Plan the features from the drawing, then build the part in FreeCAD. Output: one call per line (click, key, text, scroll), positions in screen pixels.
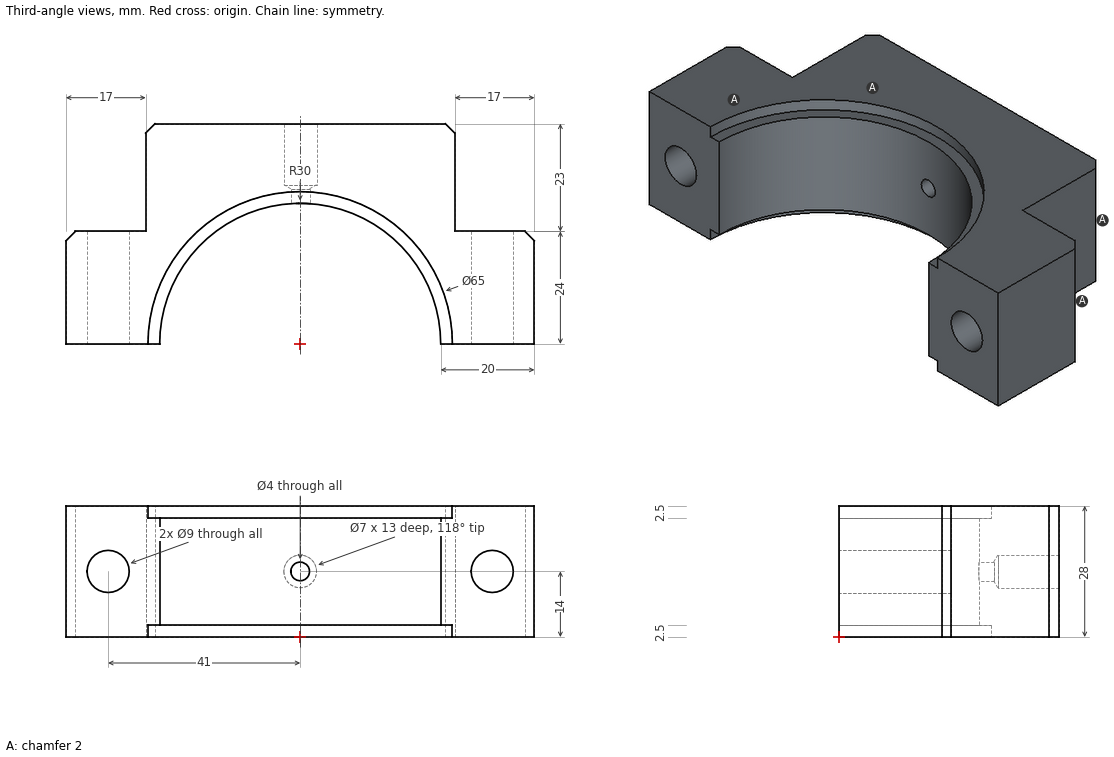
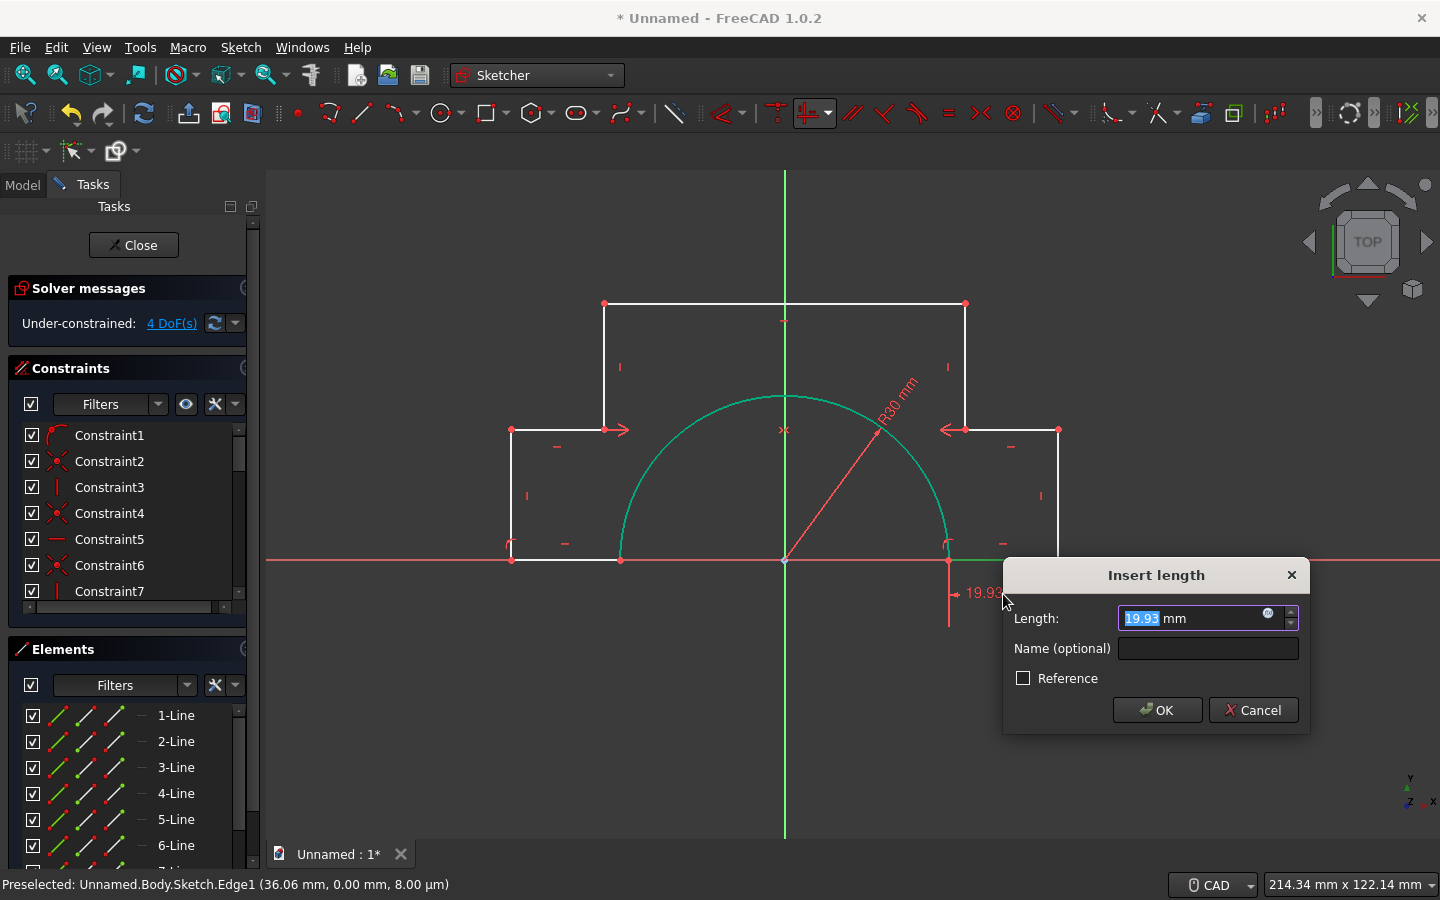
text(20)
key(Return)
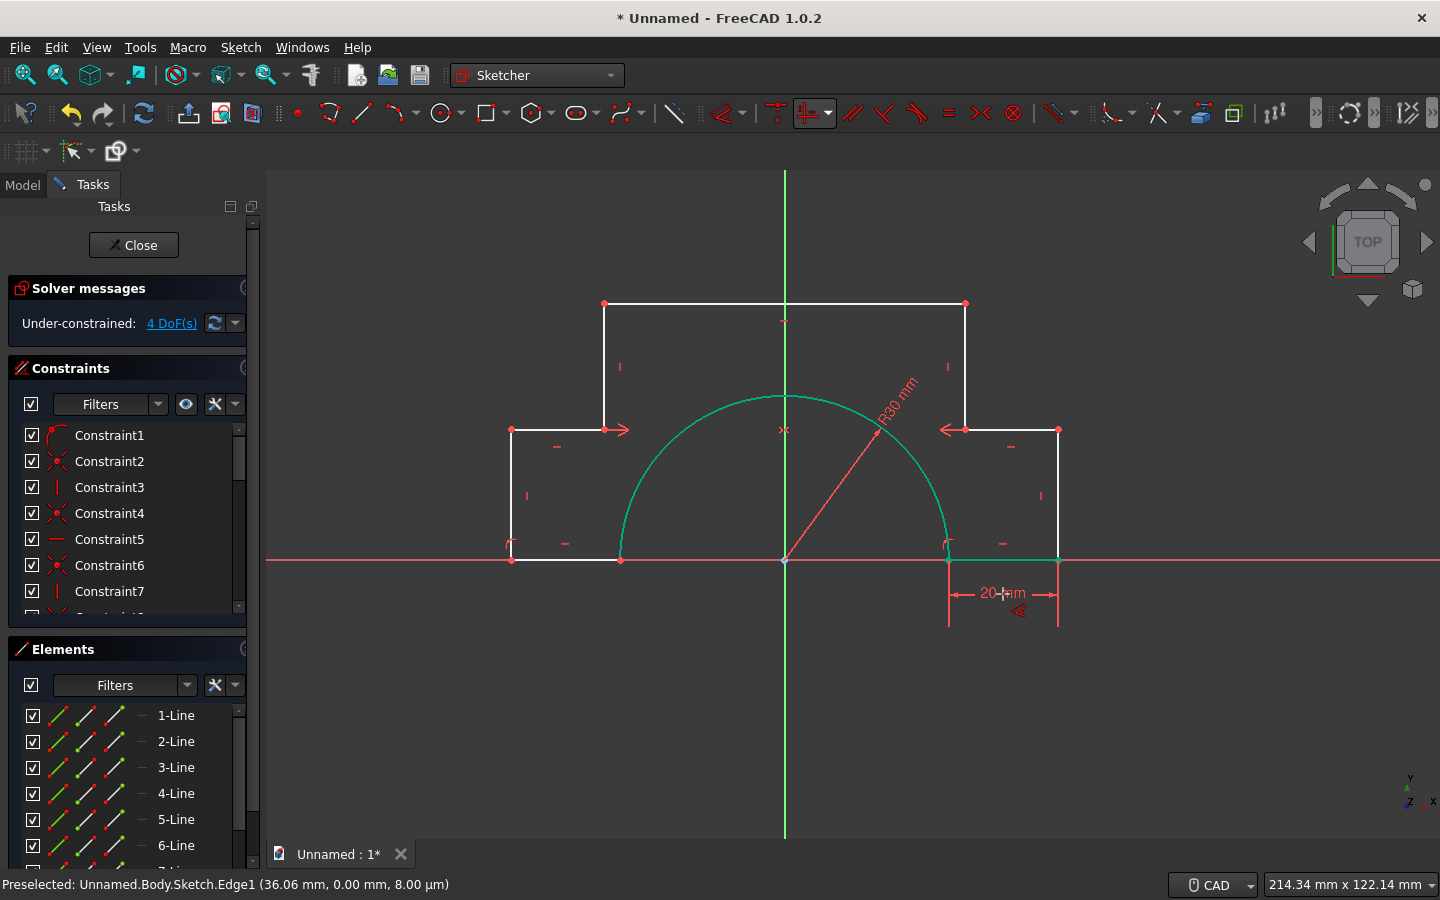
click(1058, 521)
click(1092, 495)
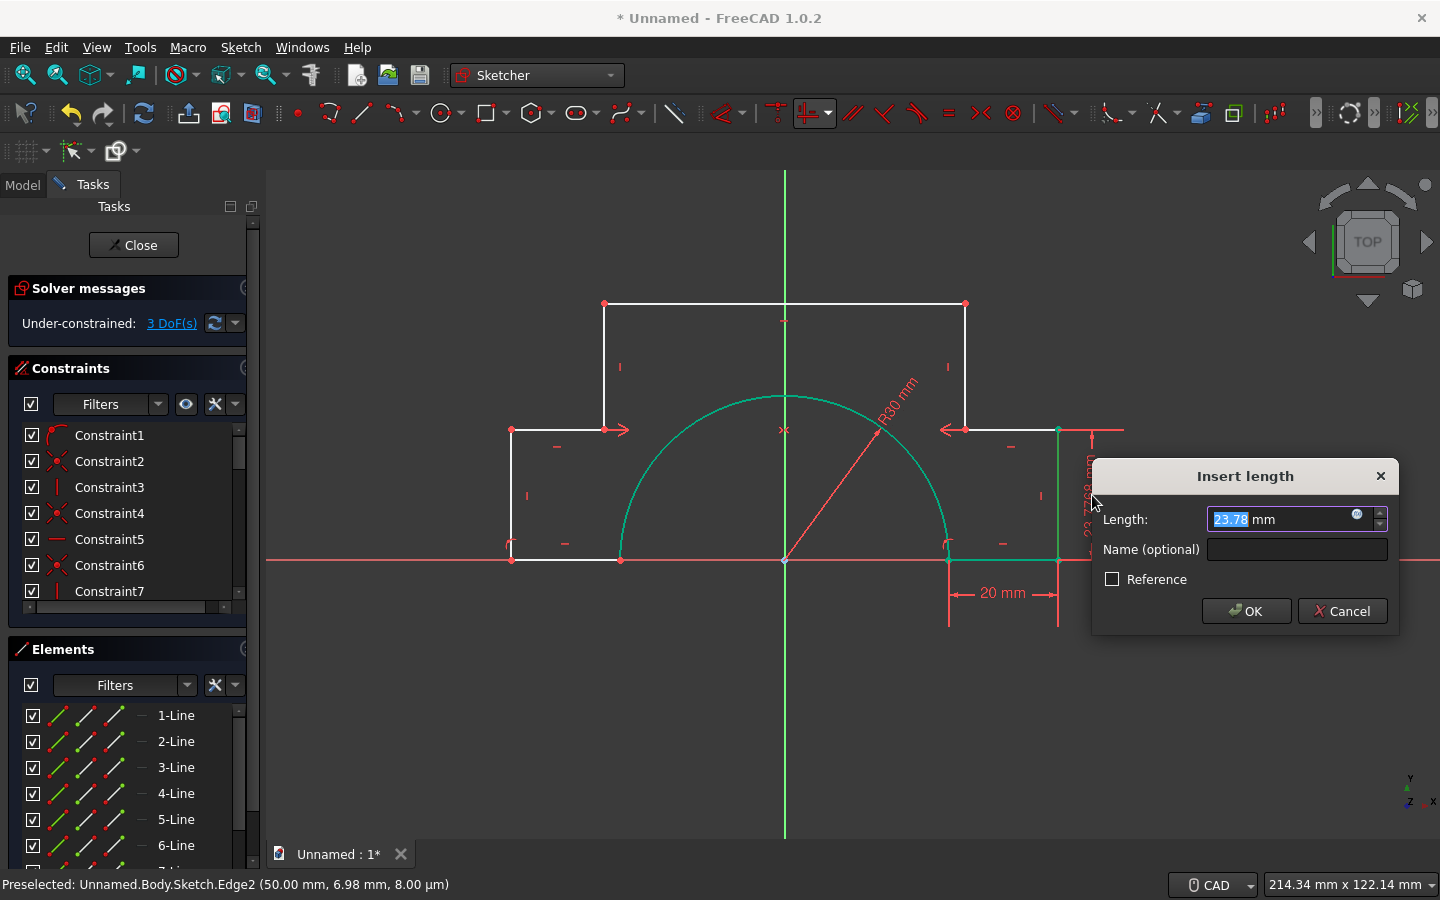
text(24)
key(Return)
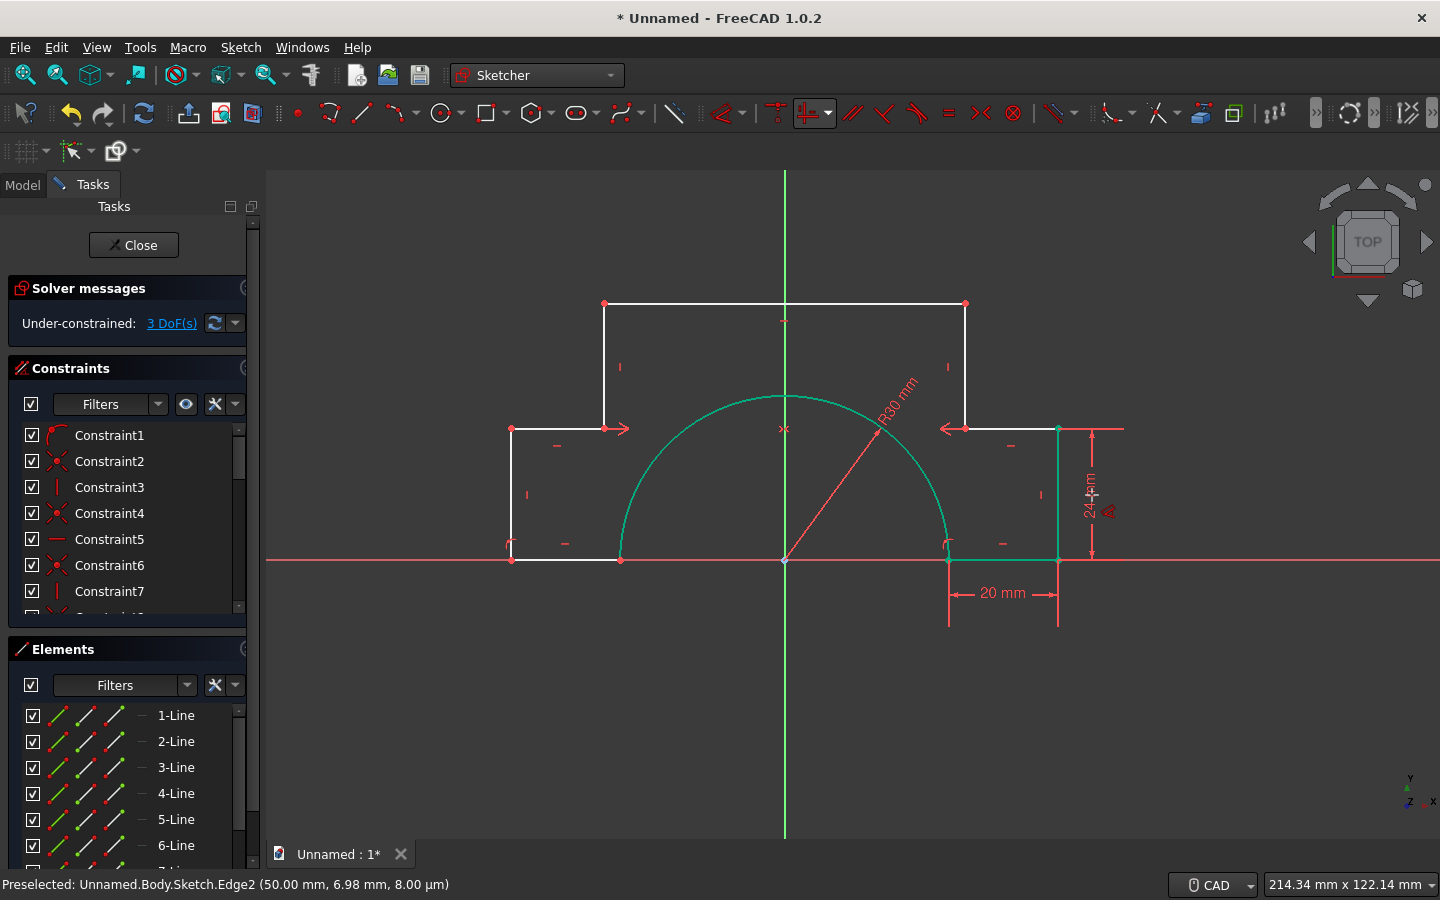
click(1030, 429)
click(1012, 395)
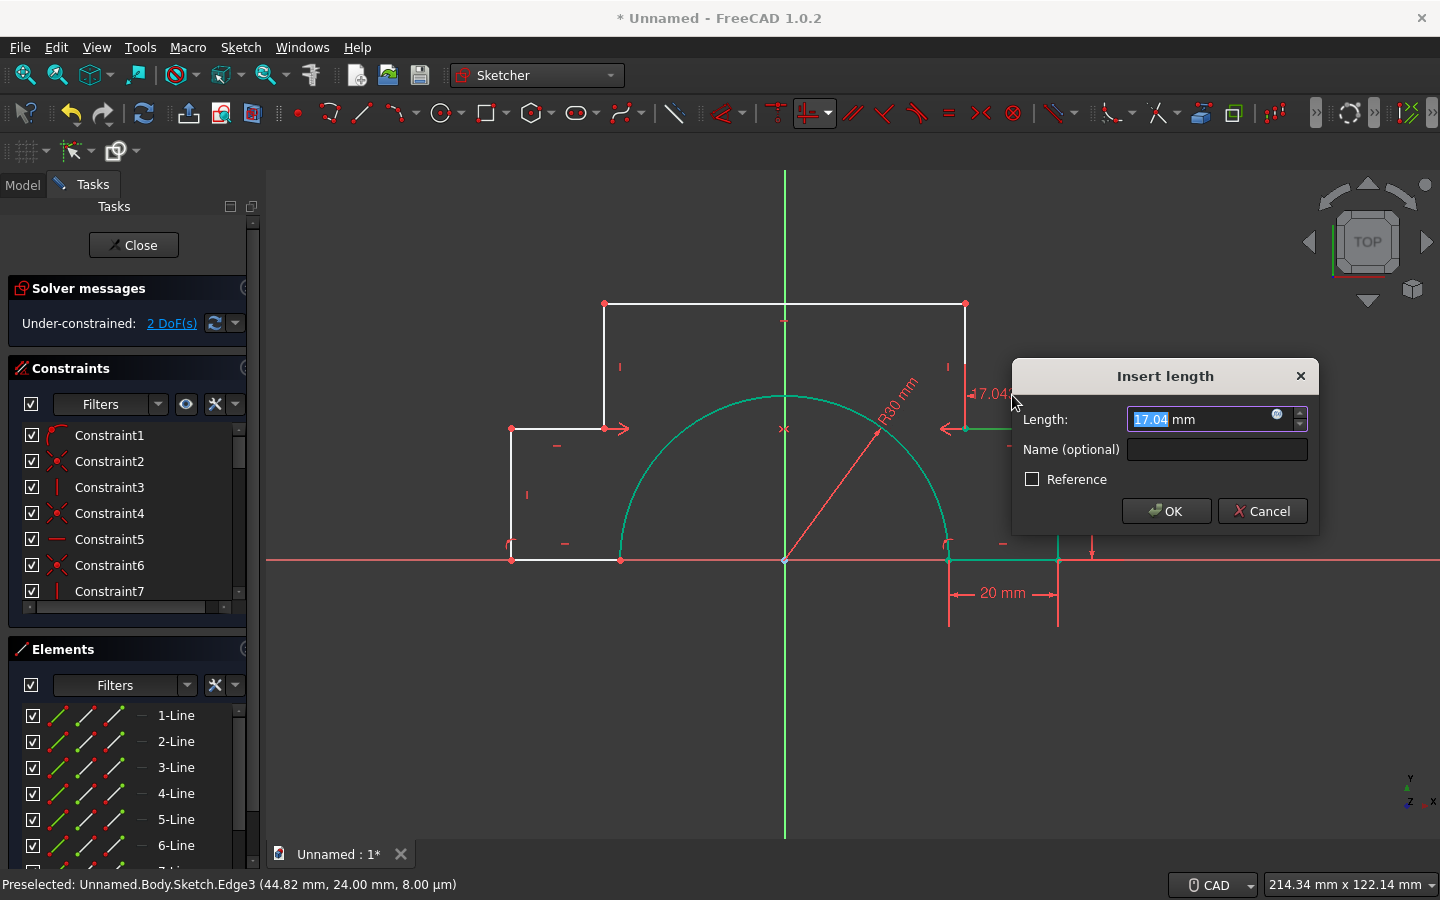
text(17)
key(Return)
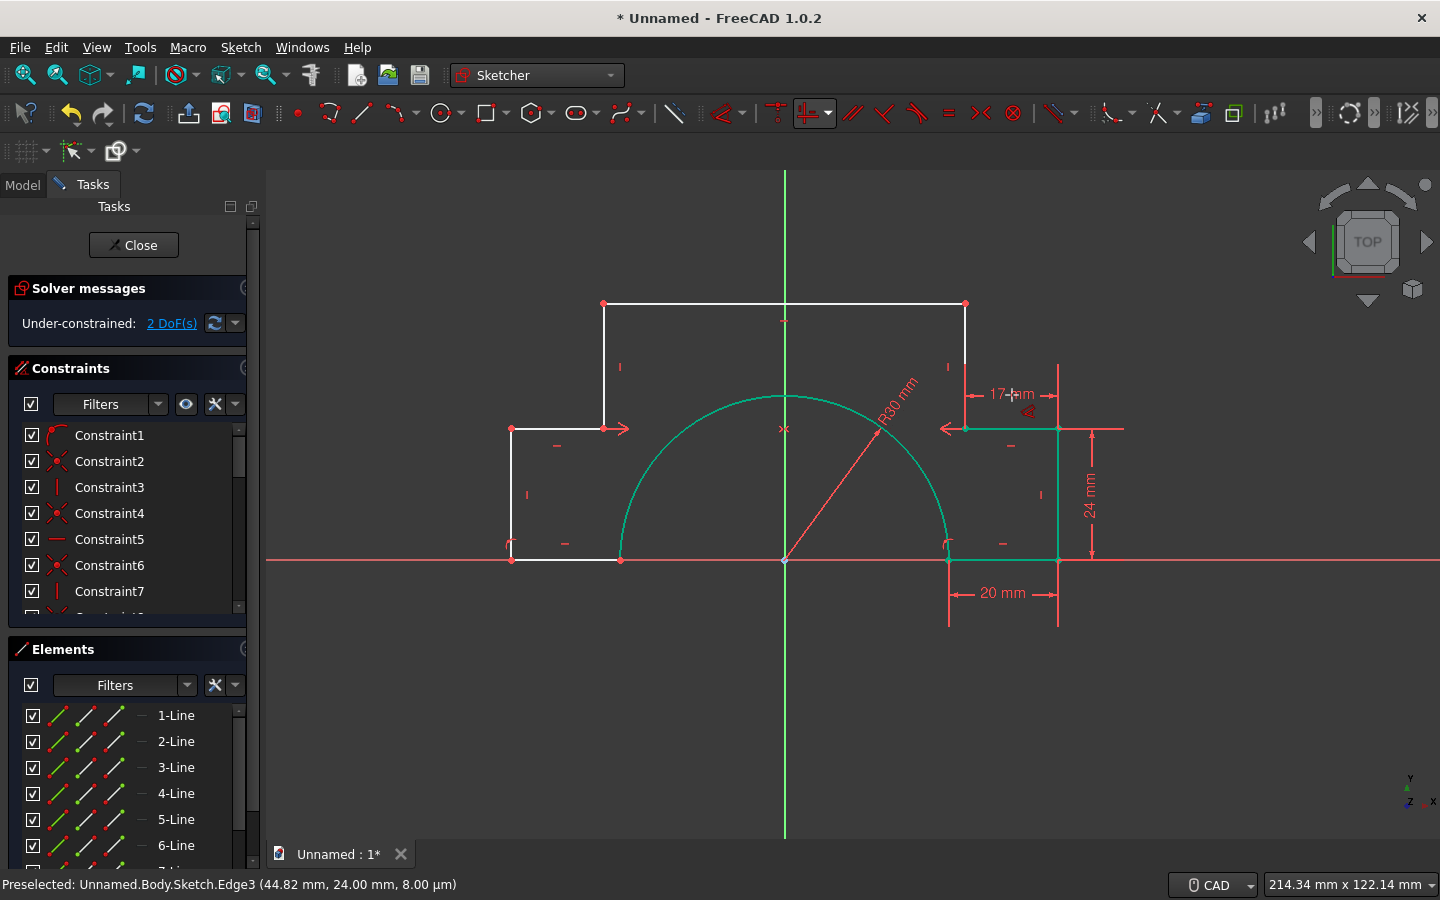
click(965, 391)
click(999, 366)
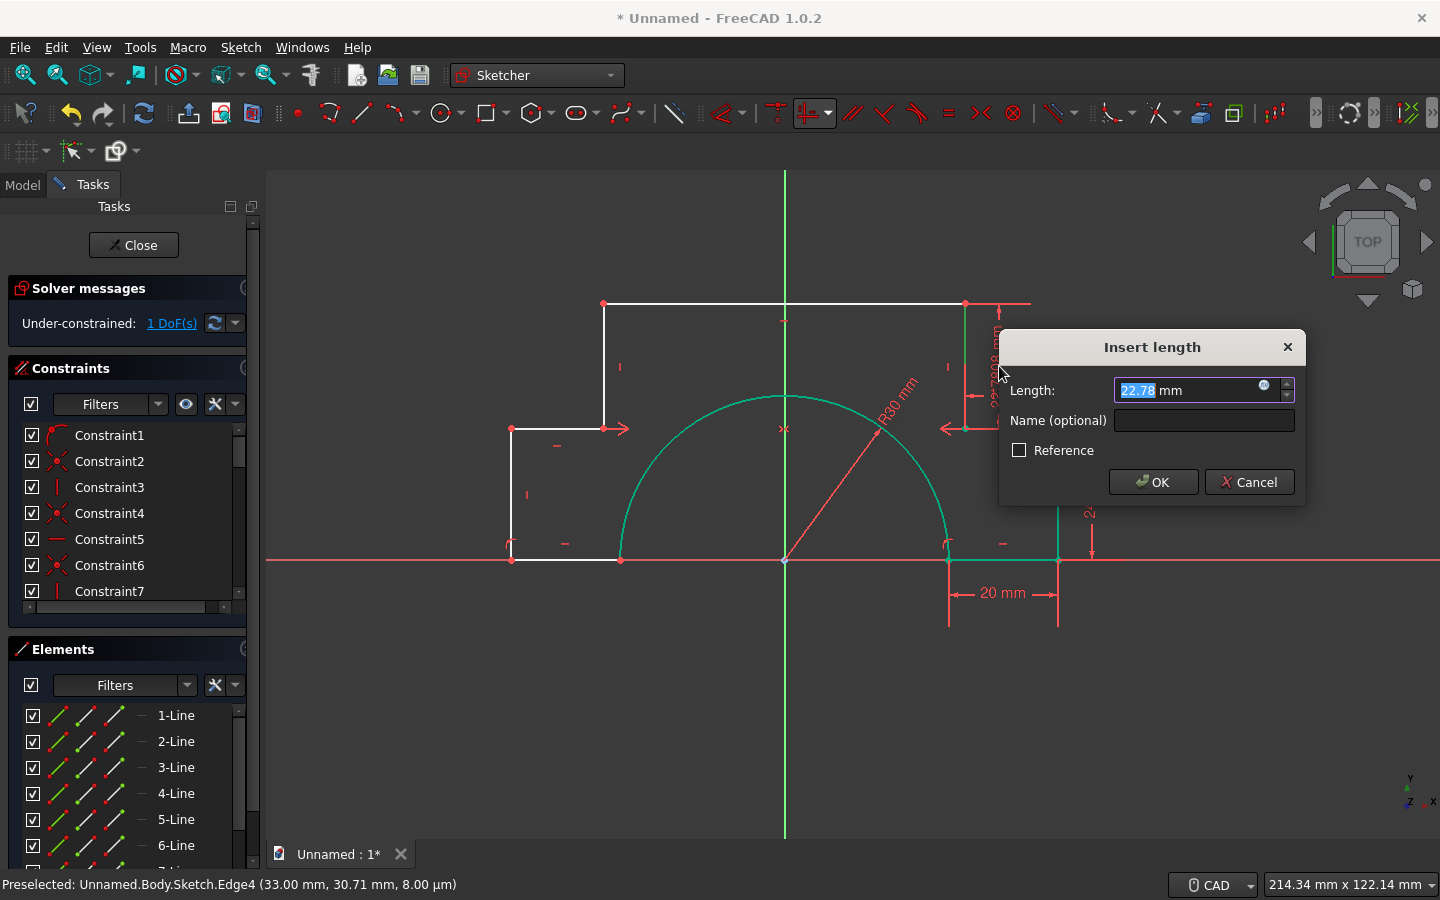
text(23)
key(Return)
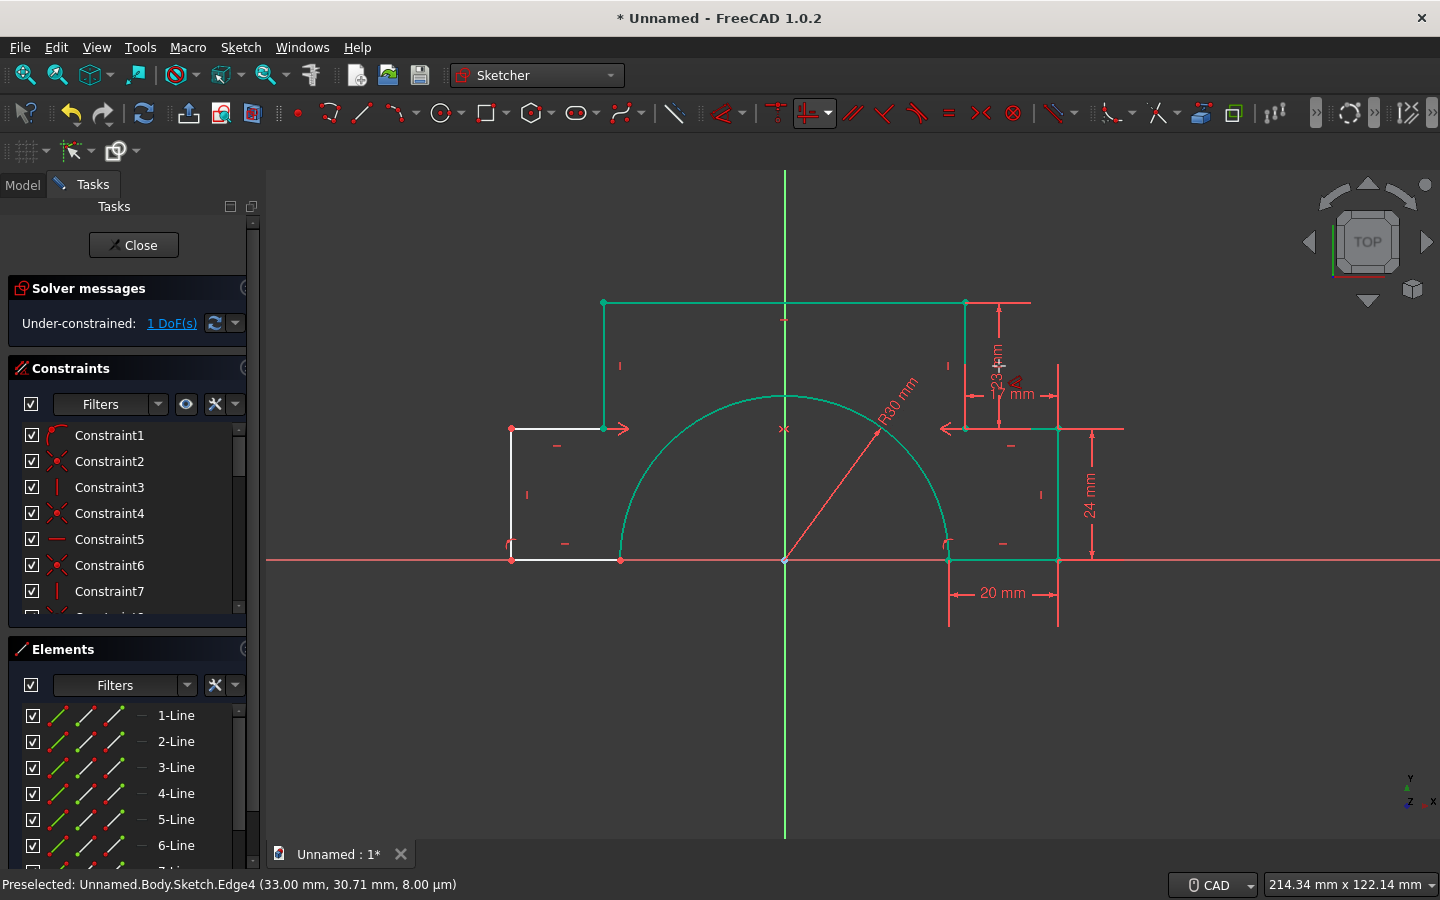
click(576, 429)
click(557, 395)